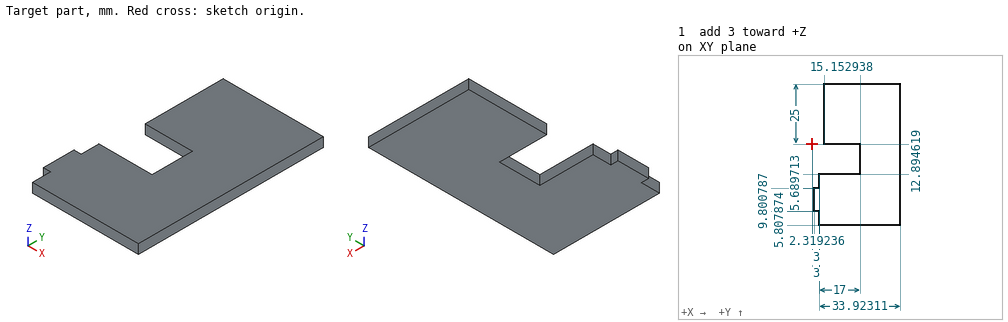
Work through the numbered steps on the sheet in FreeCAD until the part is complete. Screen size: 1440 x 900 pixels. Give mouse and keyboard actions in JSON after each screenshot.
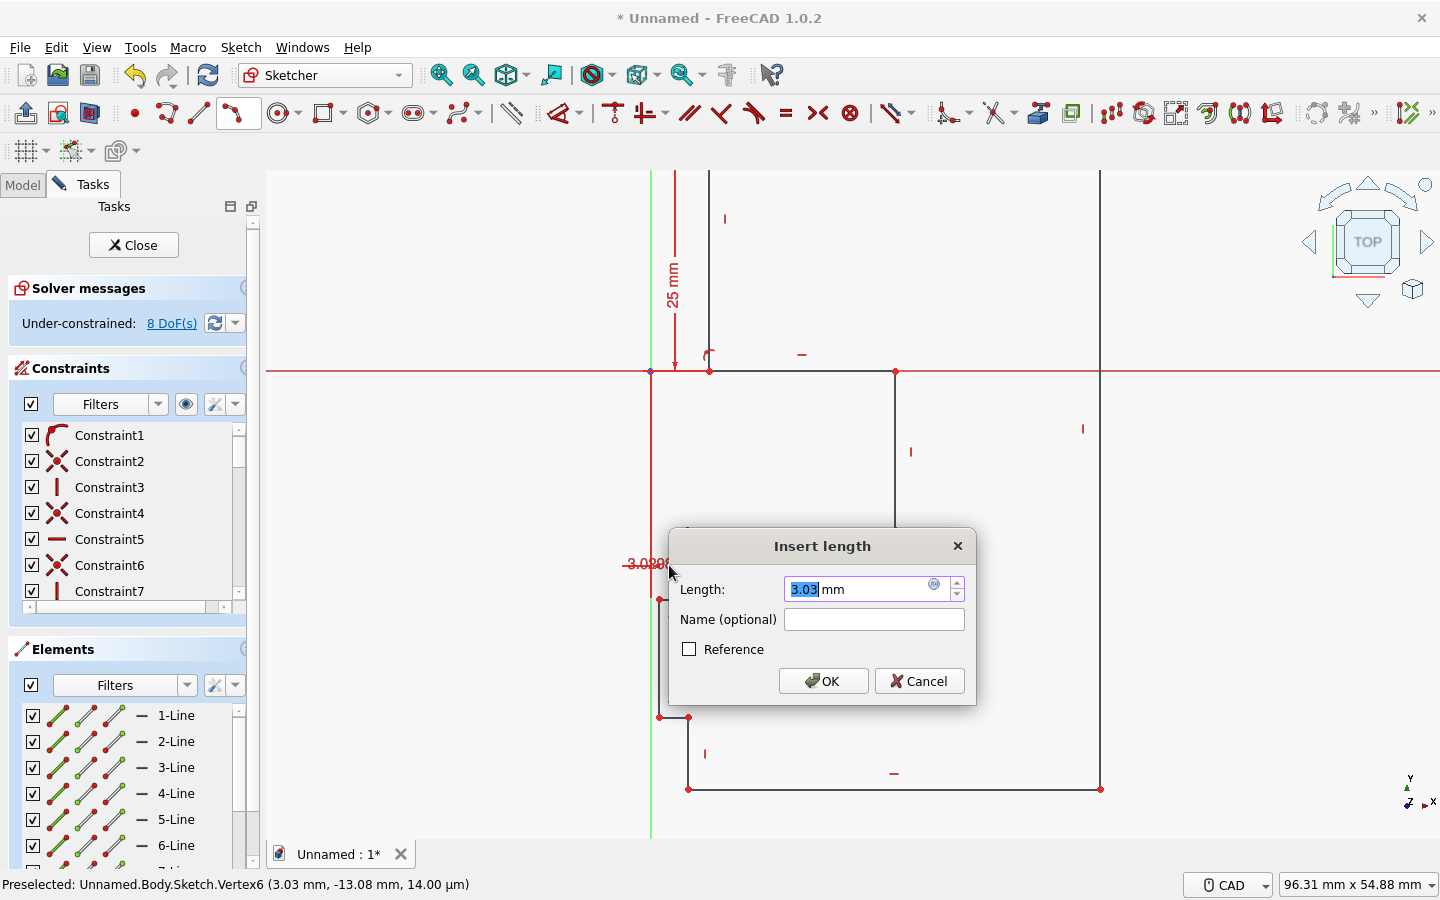
{"action": "type", "text": "3"}
{"action": "key", "text": "Return"}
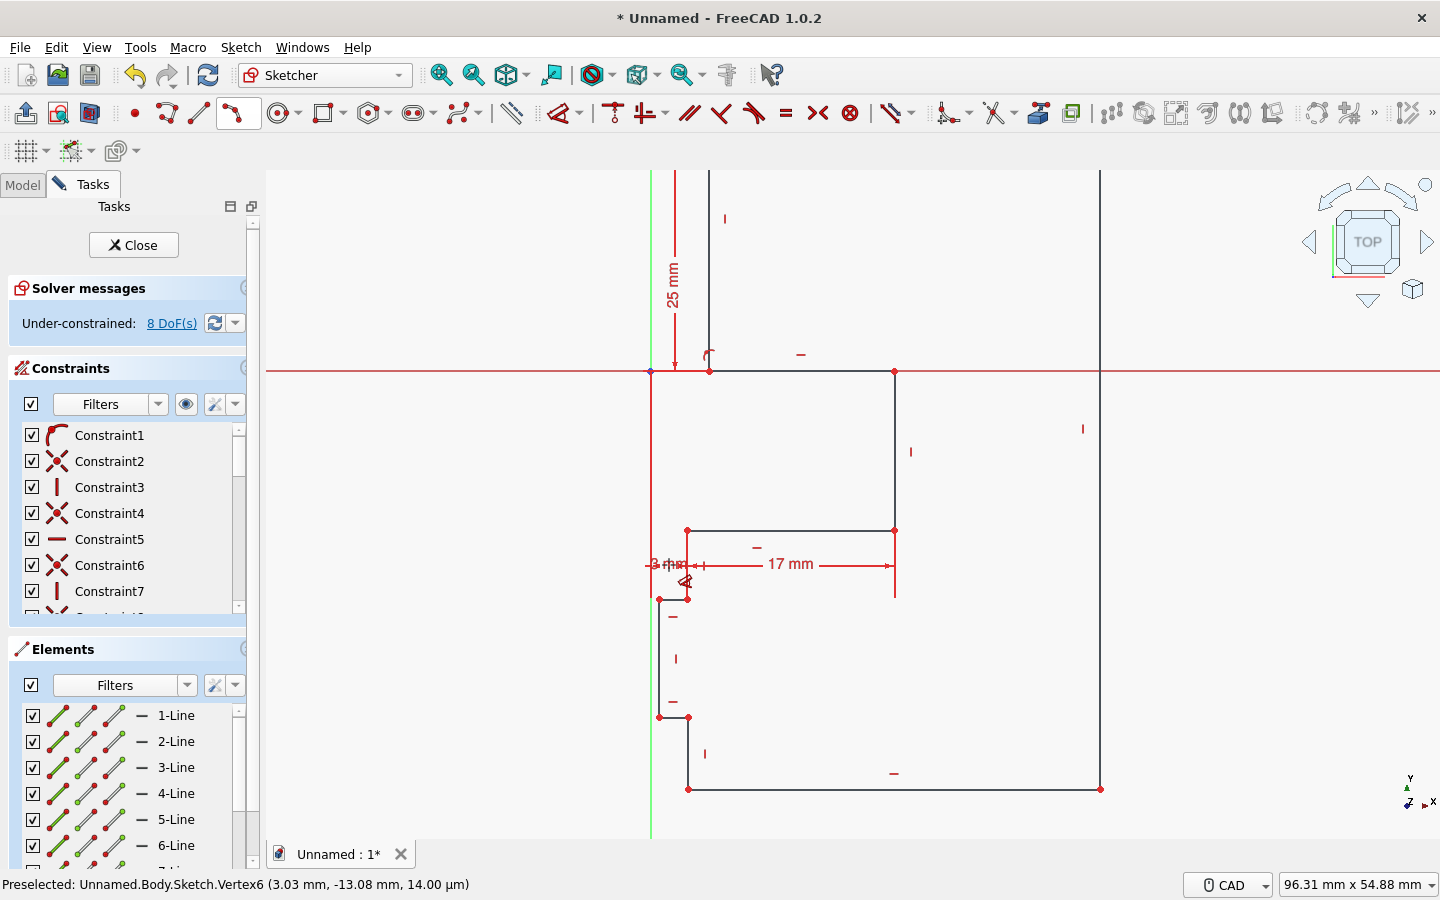
{"action": "left_click", "coordinate": [688, 718]}
{"action": "left_click", "coordinate": [670, 752]}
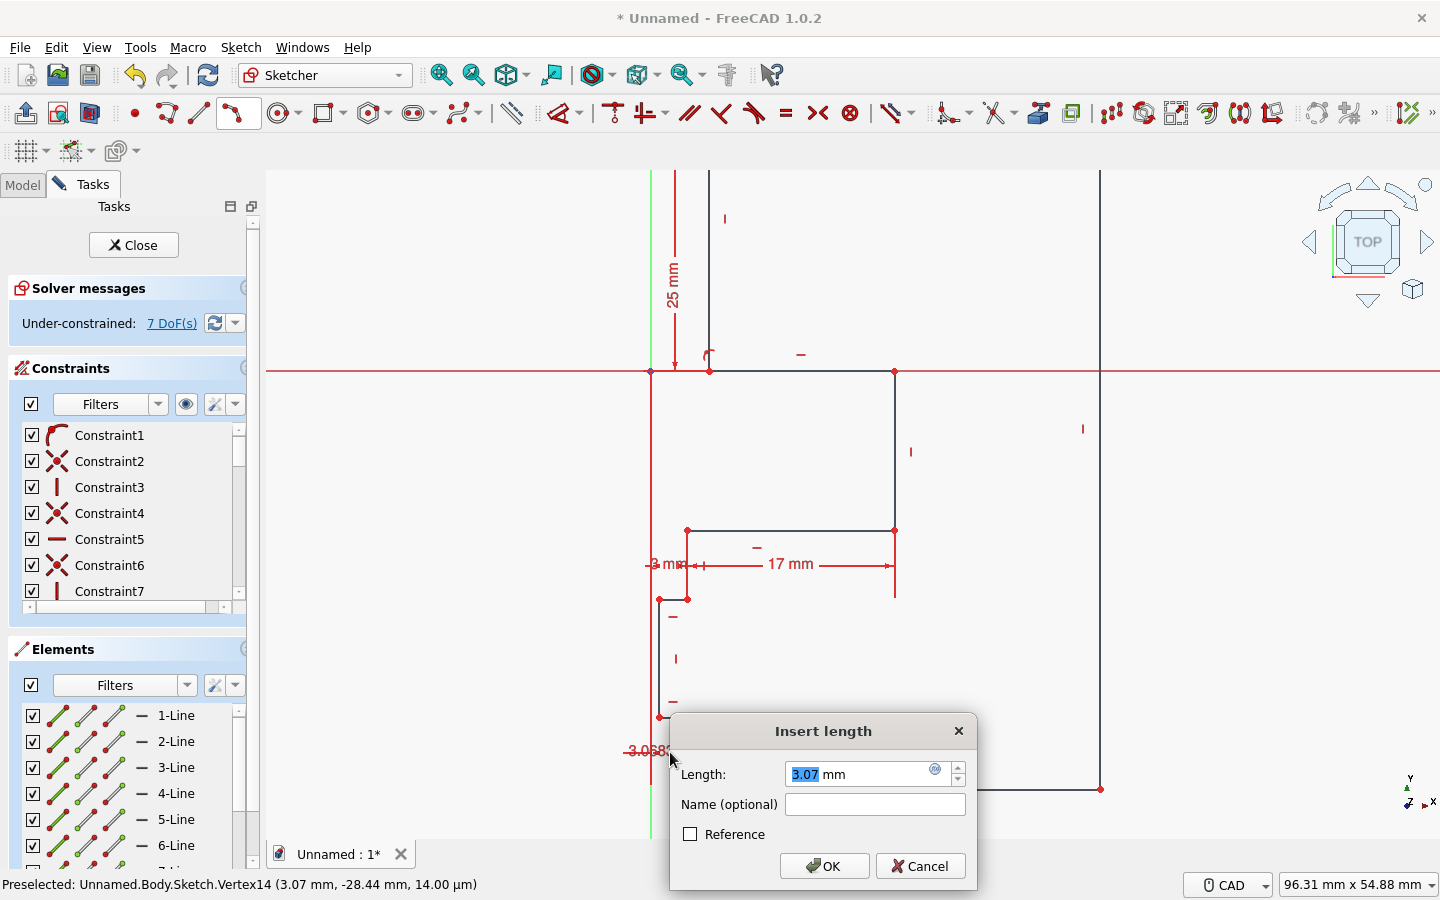
{"action": "type", "text": "3"}
{"action": "key", "text": "Return"}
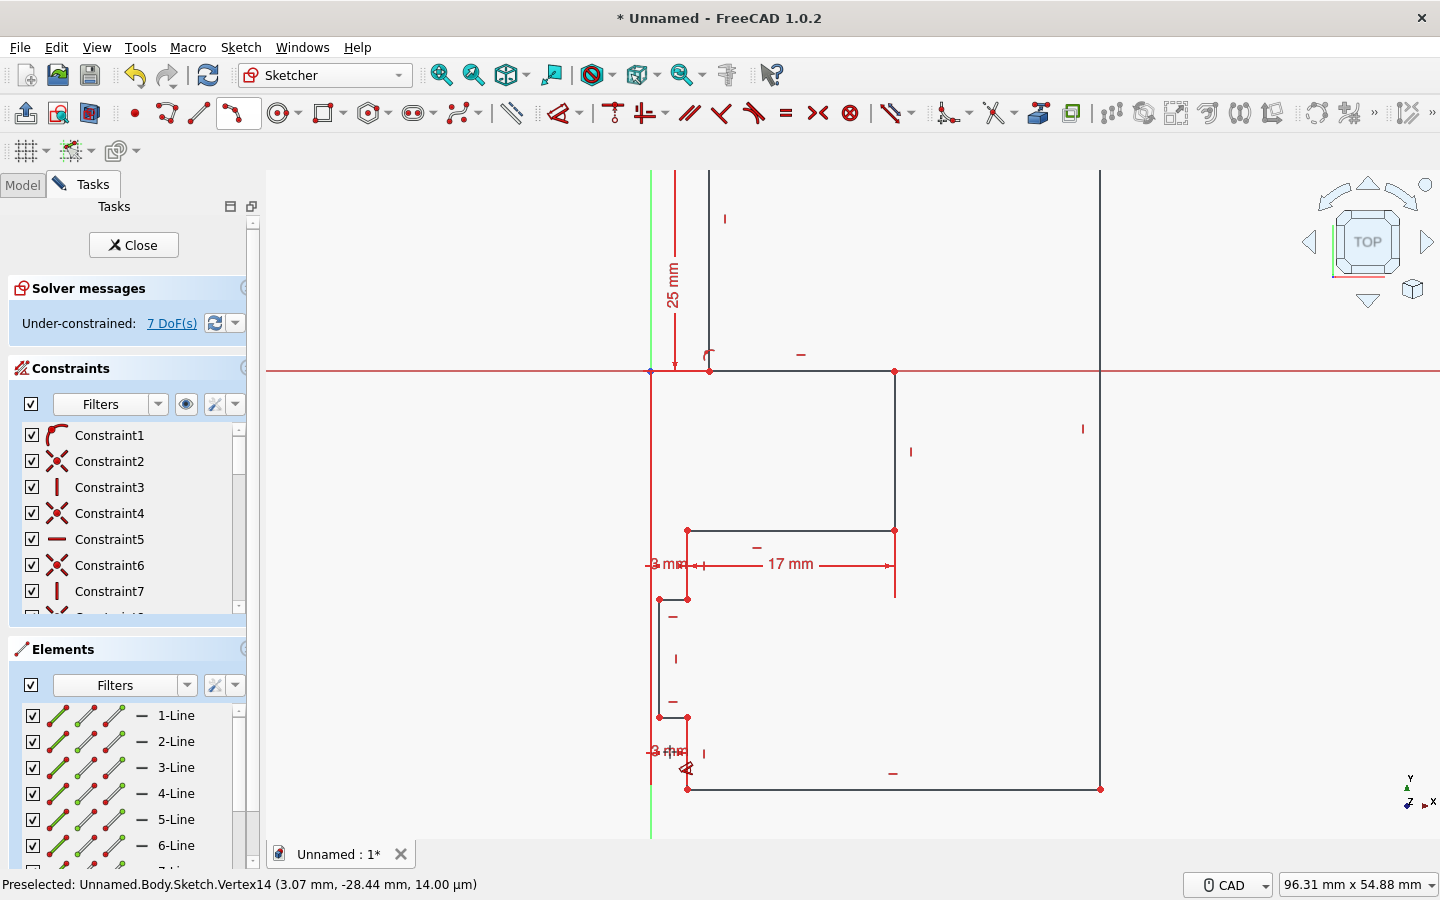
{"action": "left_click", "coordinate": [687, 551]}
{"action": "left_click", "coordinate": [721, 590]}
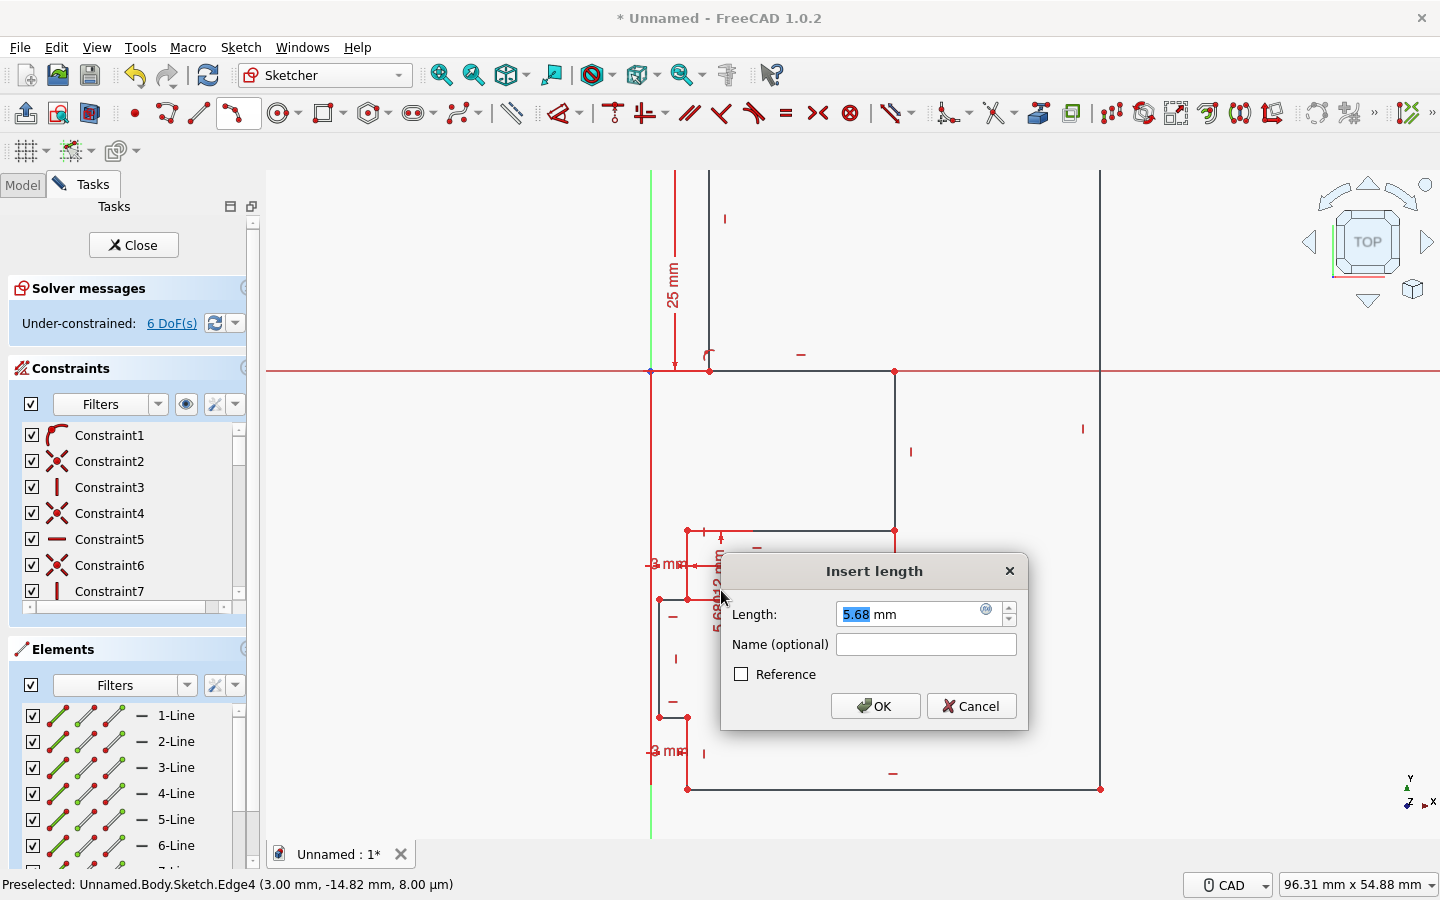
{"action": "type", "text": "5.689713"}
{"action": "key", "text": "Return"}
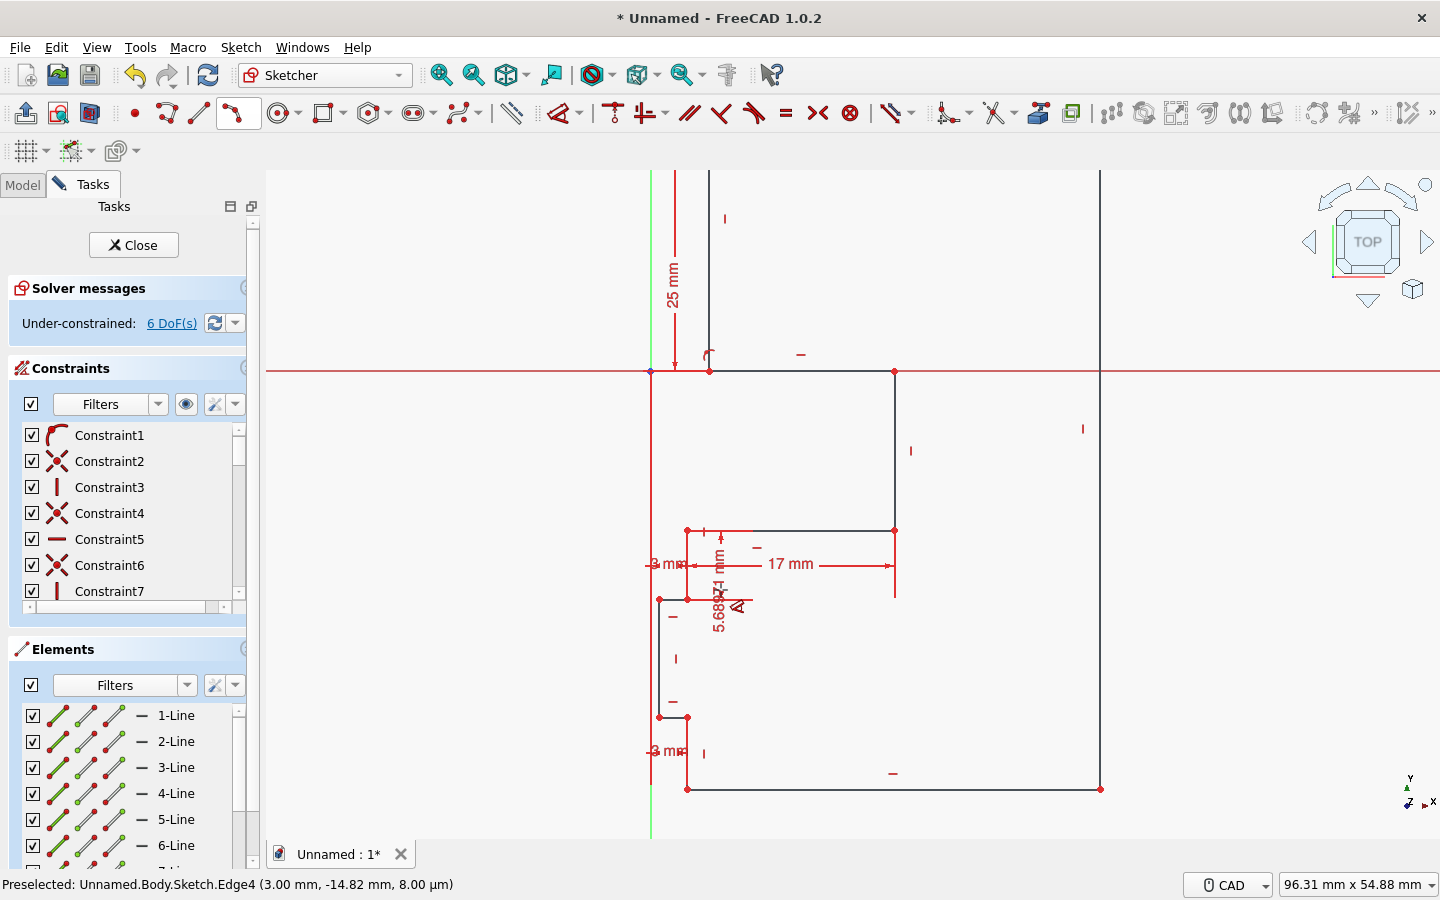
{"action": "scroll", "coordinate": [676, 600], "scroll_direction": "up", "scroll_amount": 2}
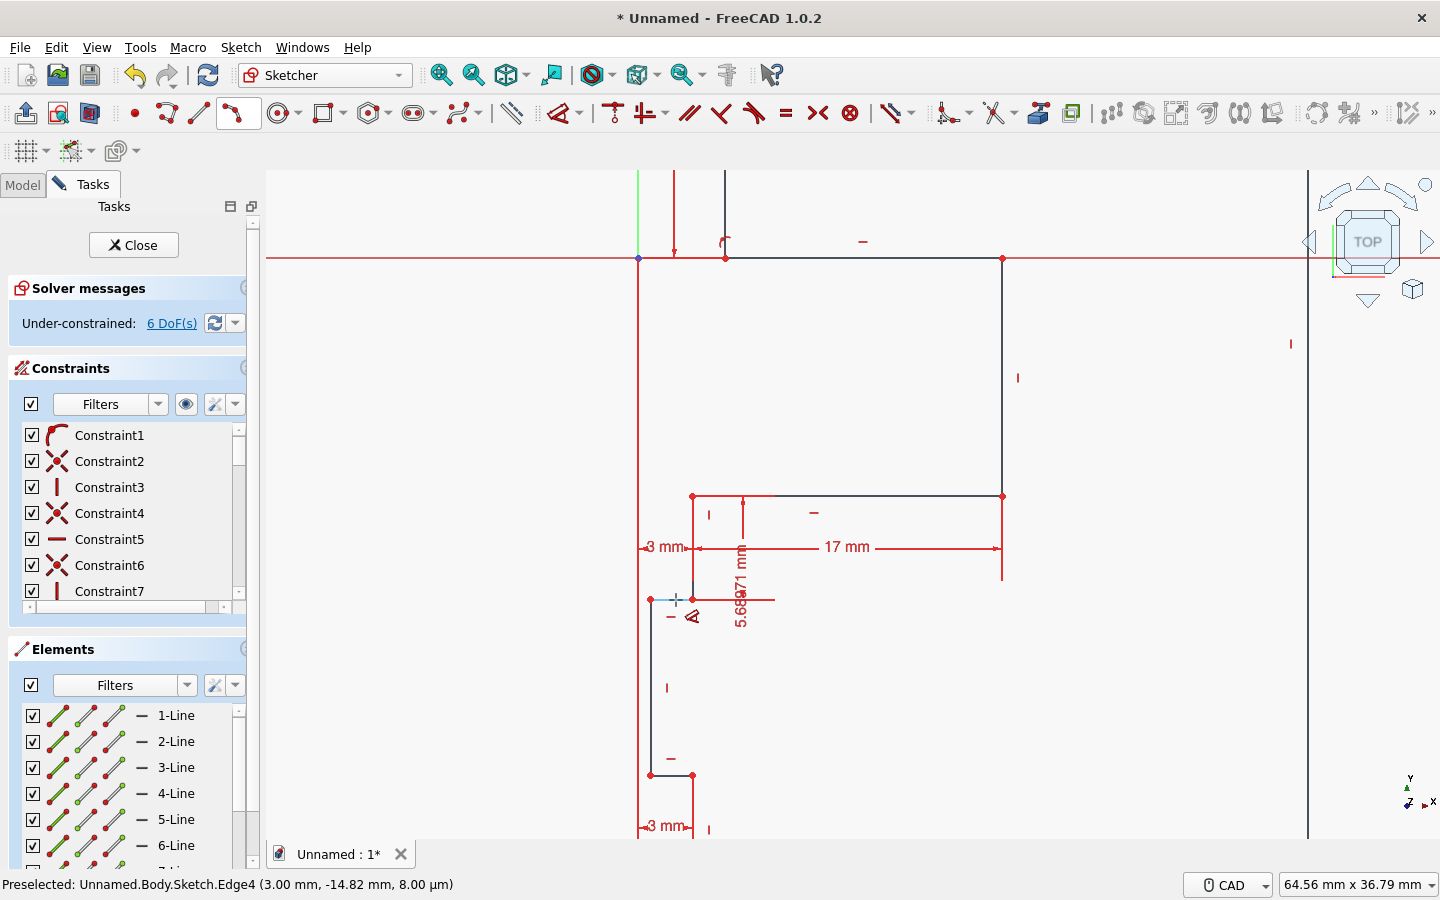
{"action": "left_click", "coordinate": [676, 600]}
{"action": "left_click", "coordinate": [672, 634]}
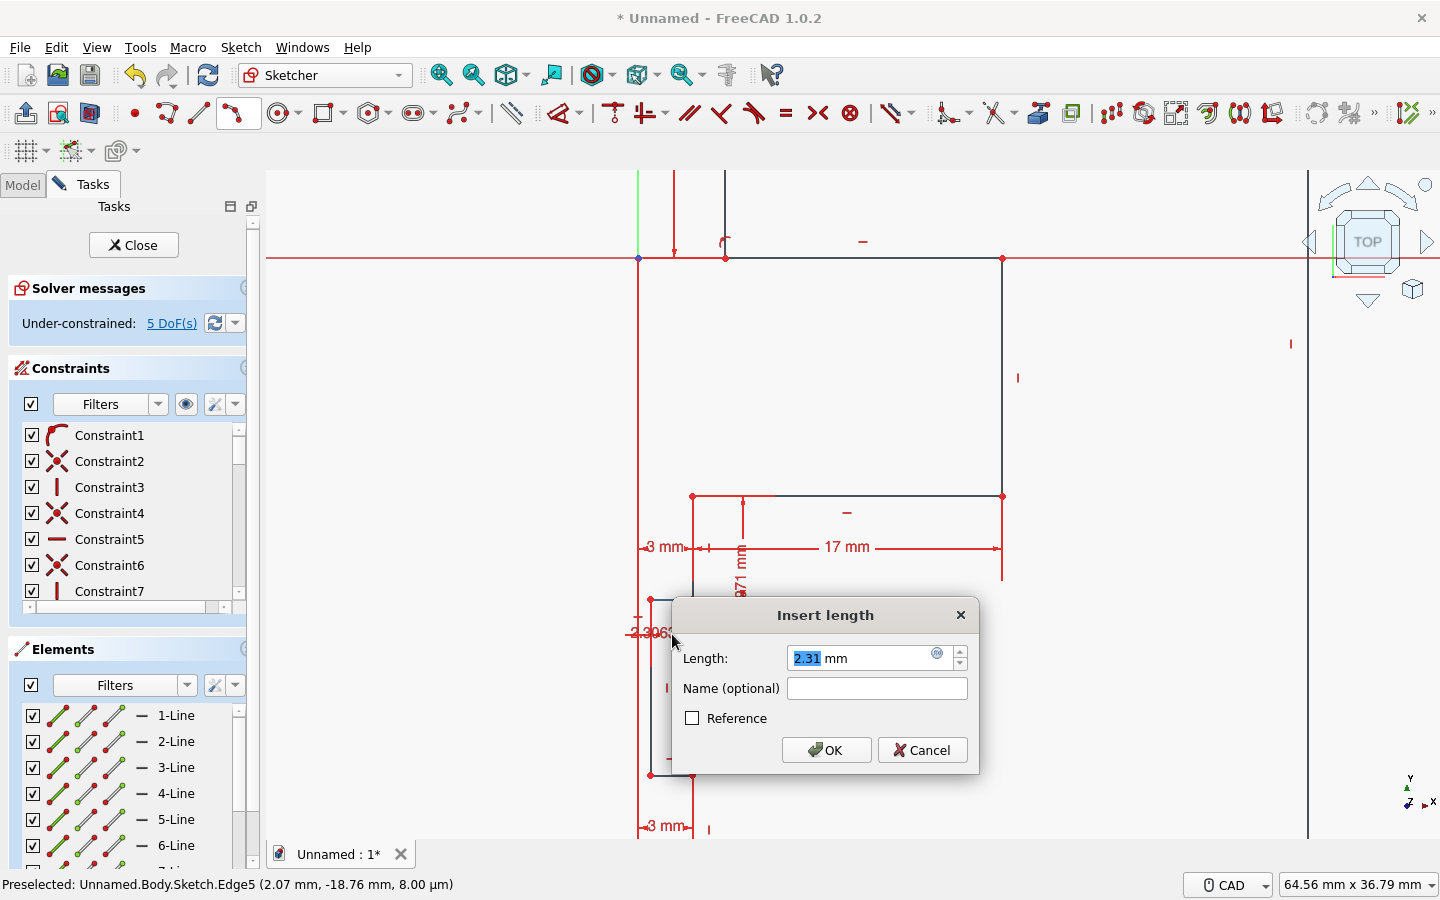
{"action": "type", "text": "2.319236"}
{"action": "key", "text": "Return"}